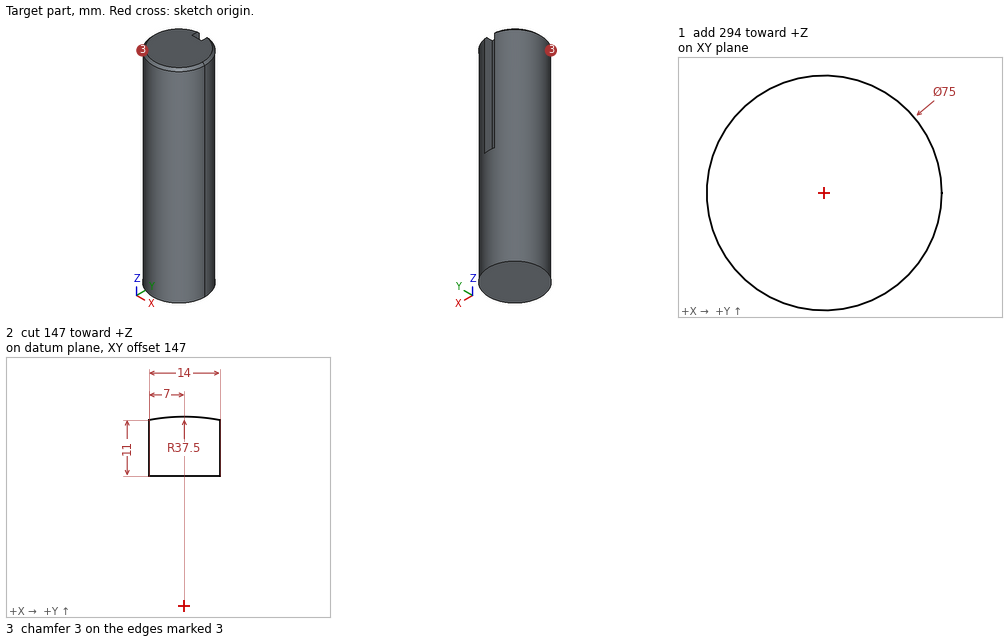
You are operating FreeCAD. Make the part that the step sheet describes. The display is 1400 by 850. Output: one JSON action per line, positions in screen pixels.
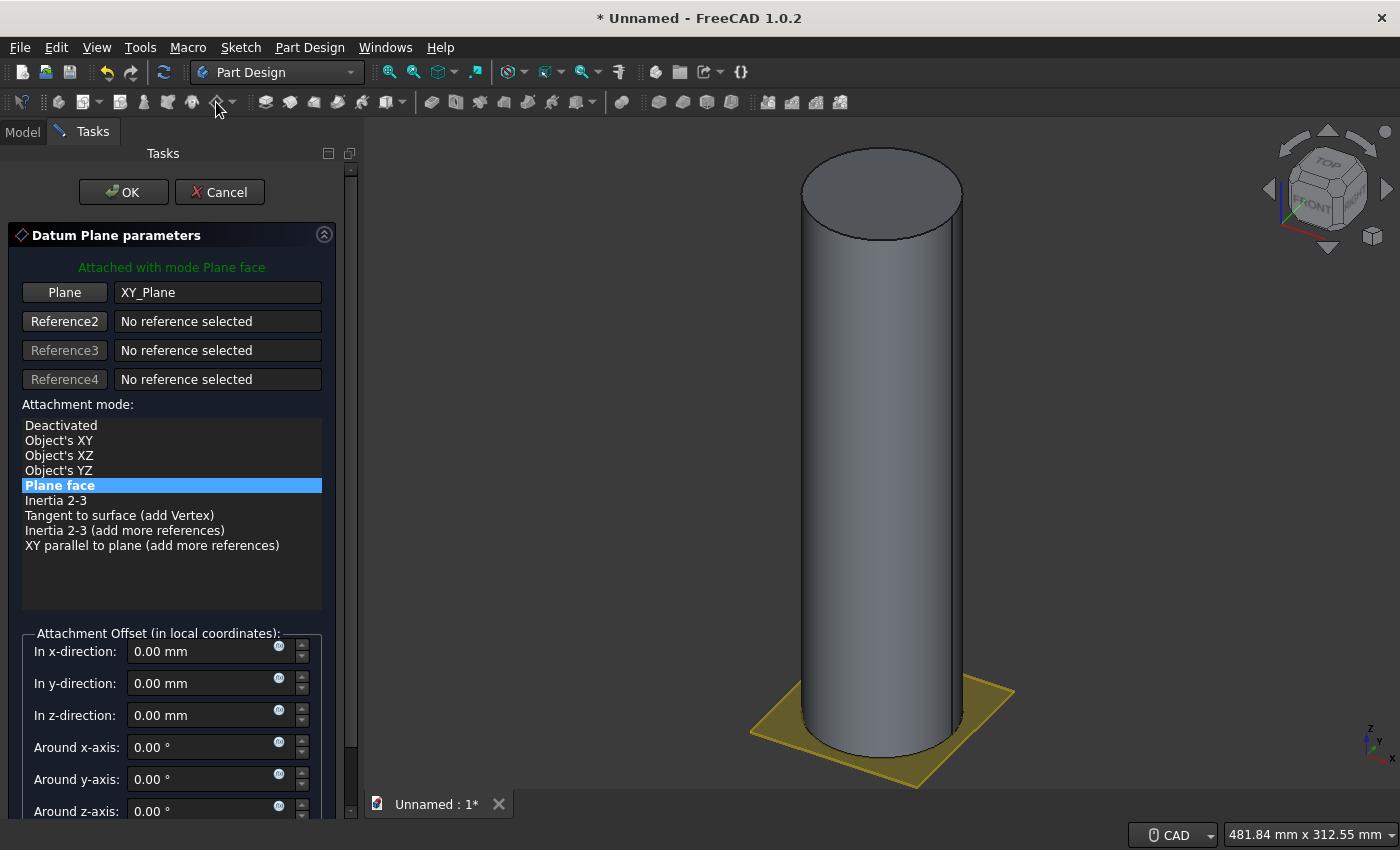
{"action": "triple_click", "coordinate": [210, 715]}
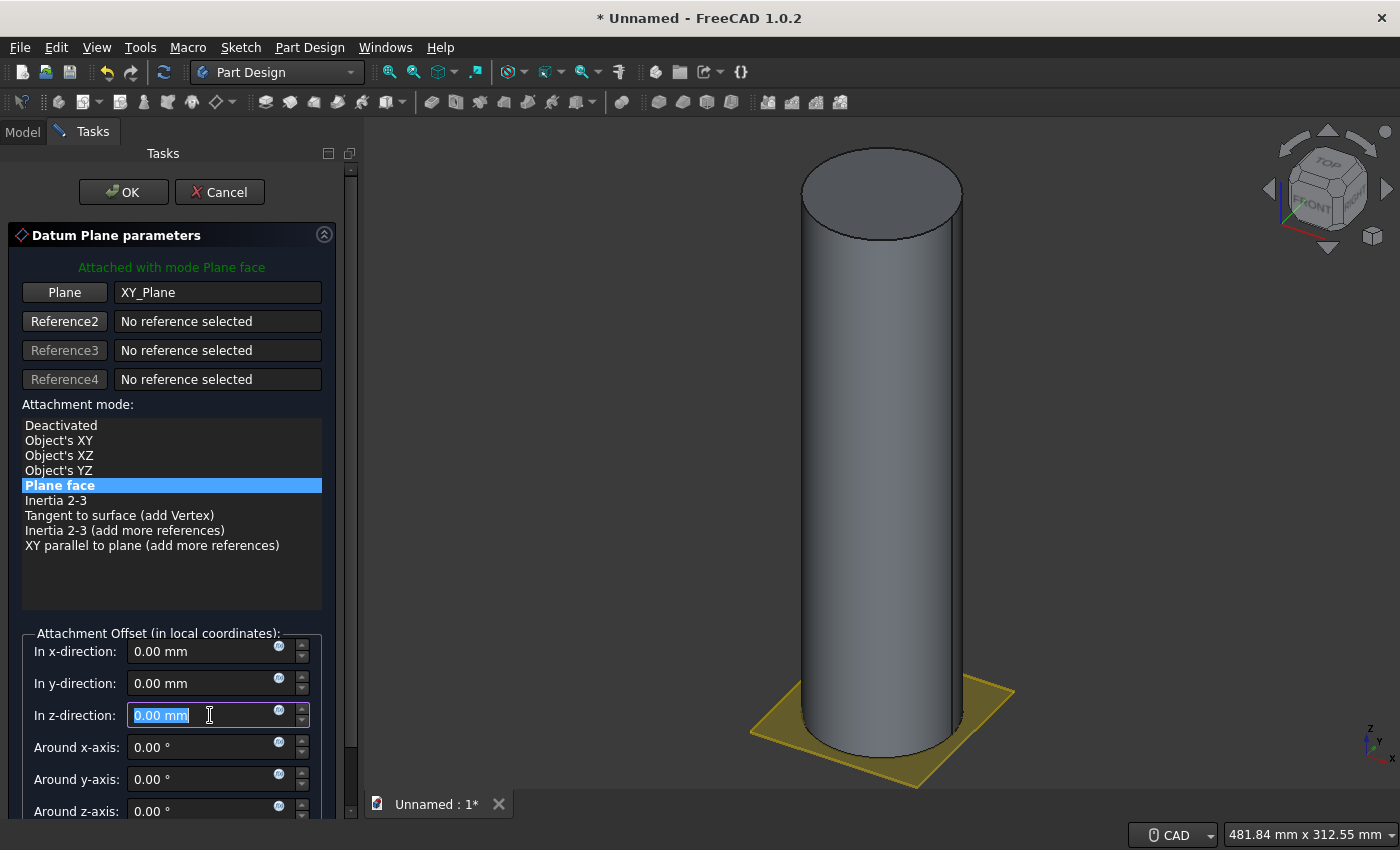
{"action": "type", "text": "147"}
{"action": "key", "text": "Tab"}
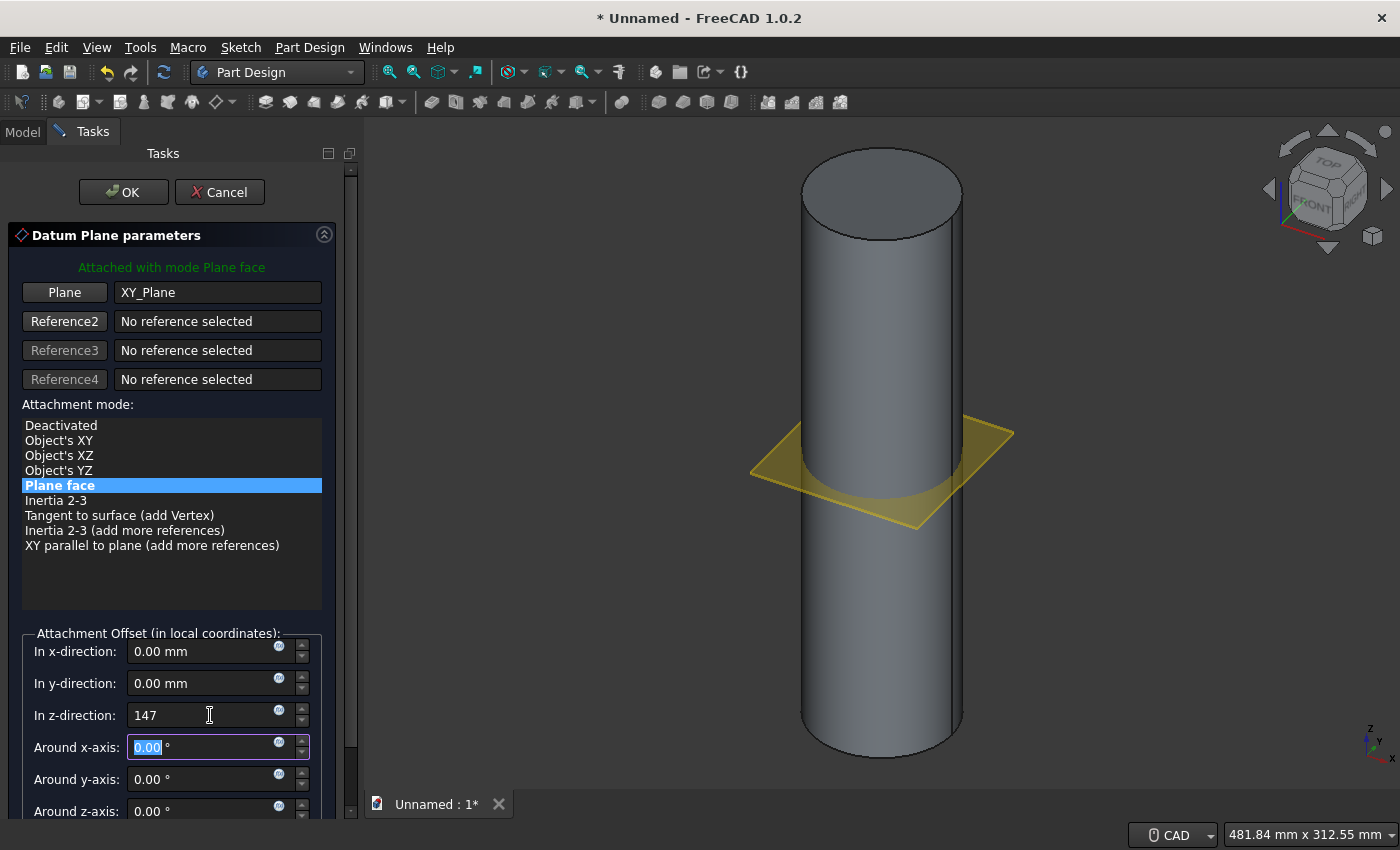
{"action": "left_click", "coordinate": [124, 192]}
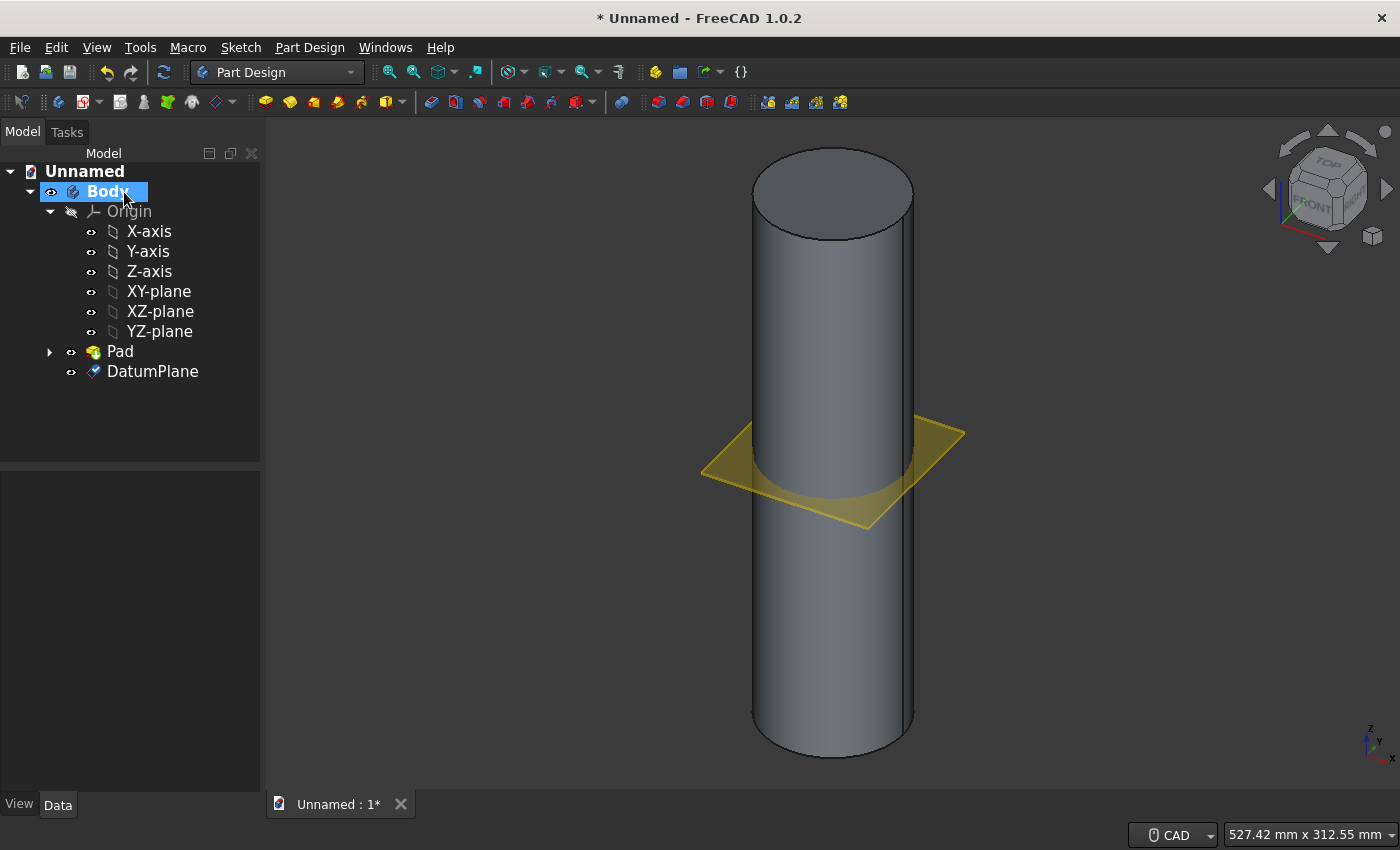
{"action": "left_click", "coordinate": [116, 372]}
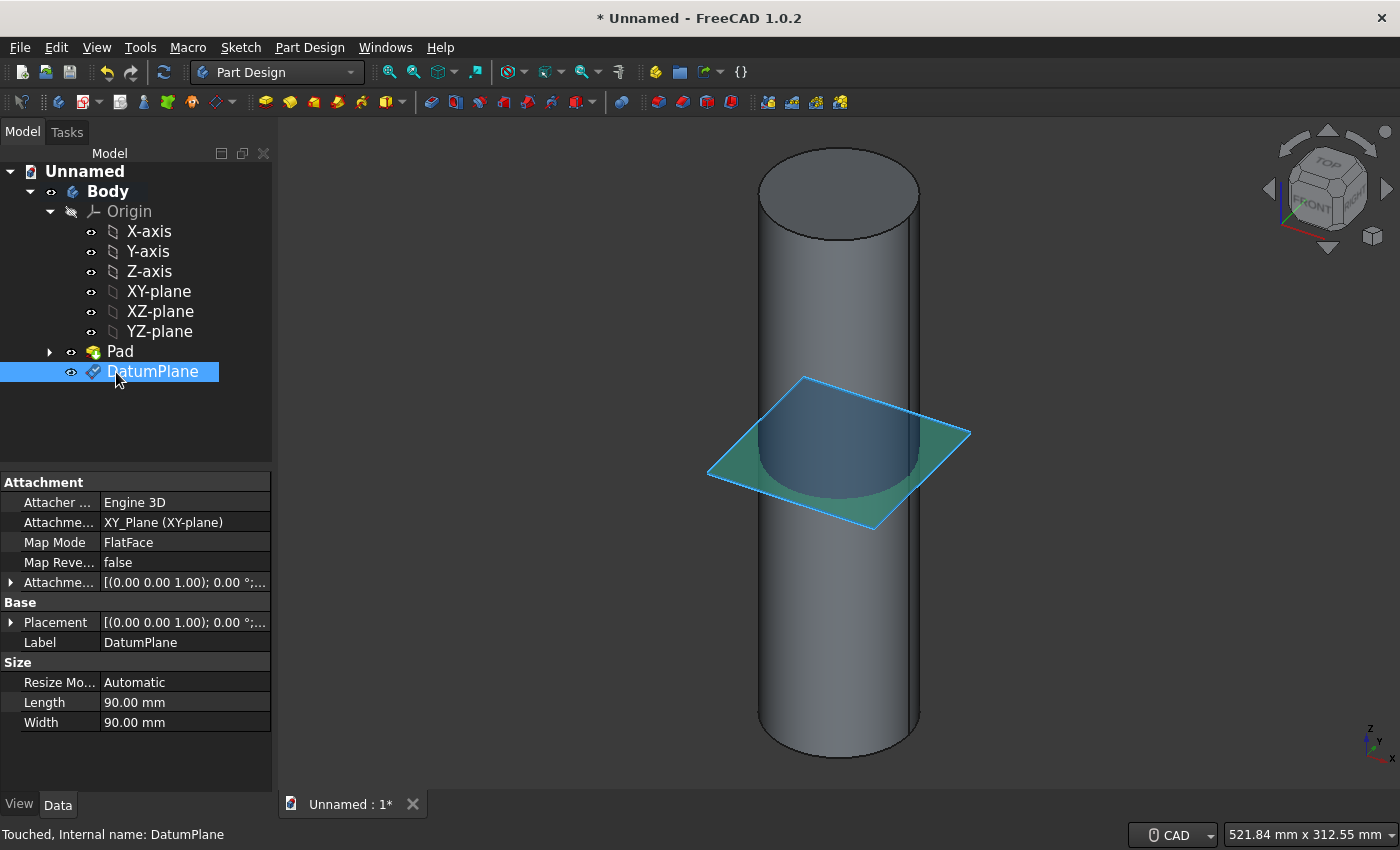
{"action": "left_click", "coordinate": [84, 102]}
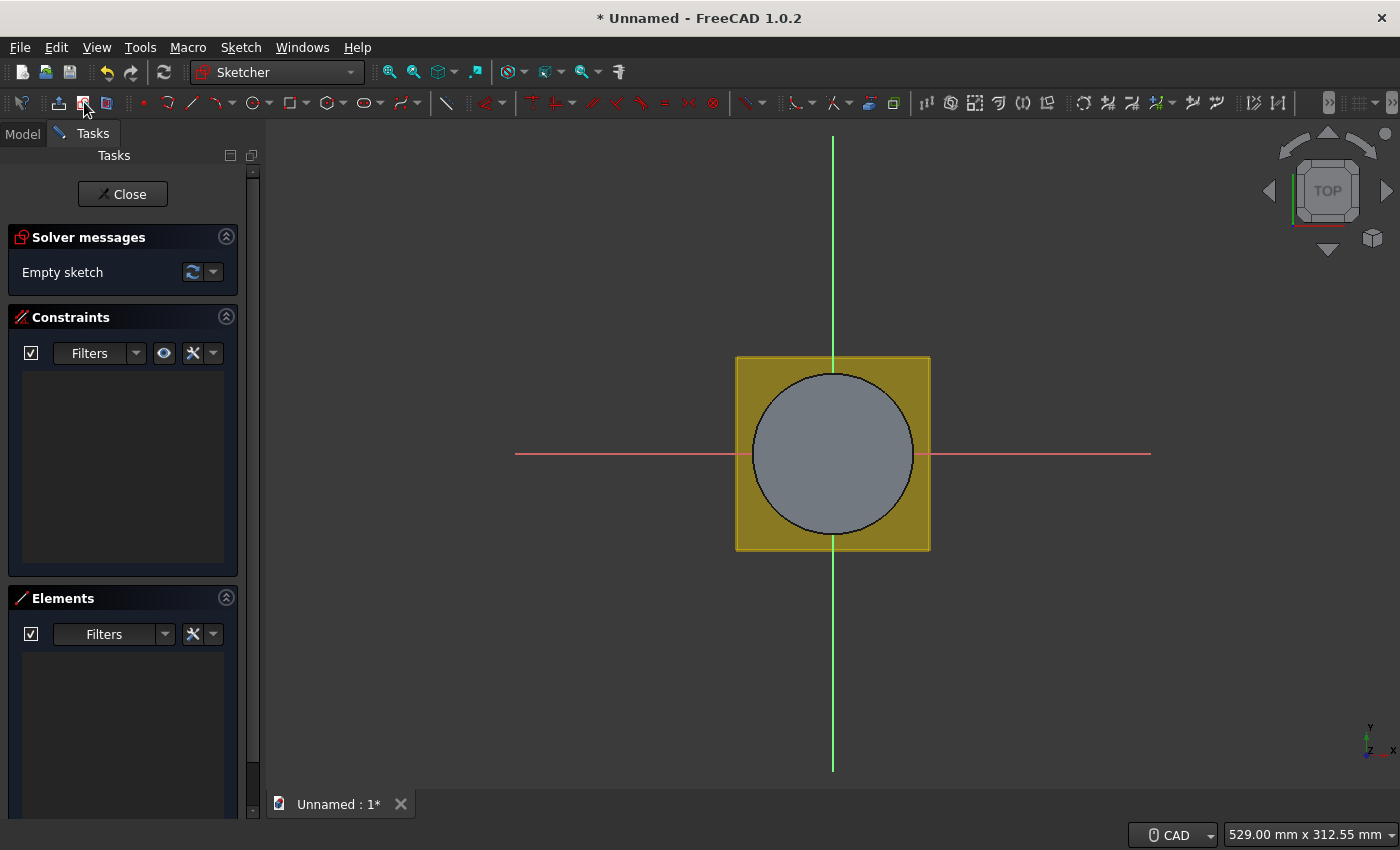
{"action": "key", "text": "q s"}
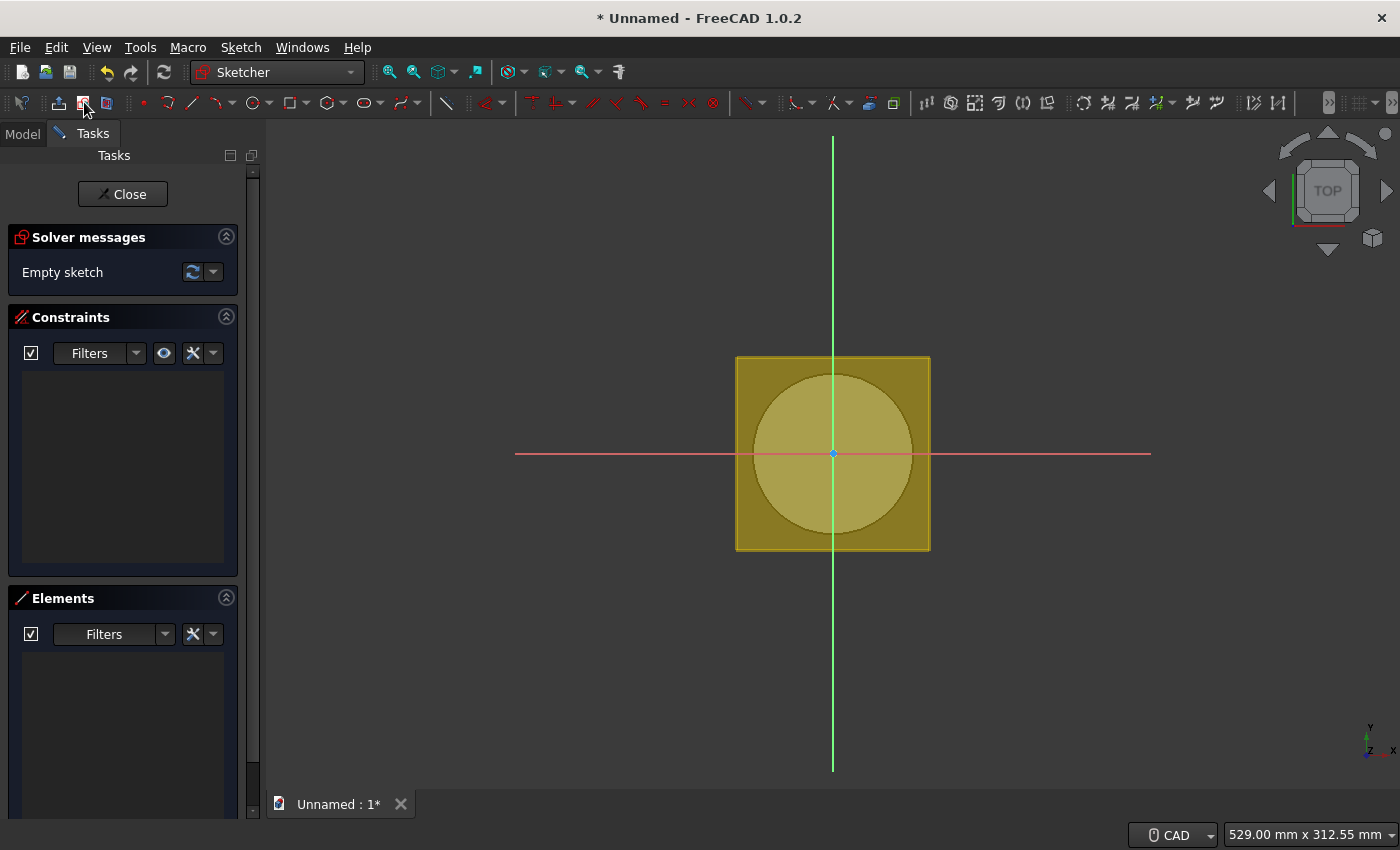
{"action": "scroll", "coordinate": [837, 382], "scroll_direction": "up", "scroll_amount": 14}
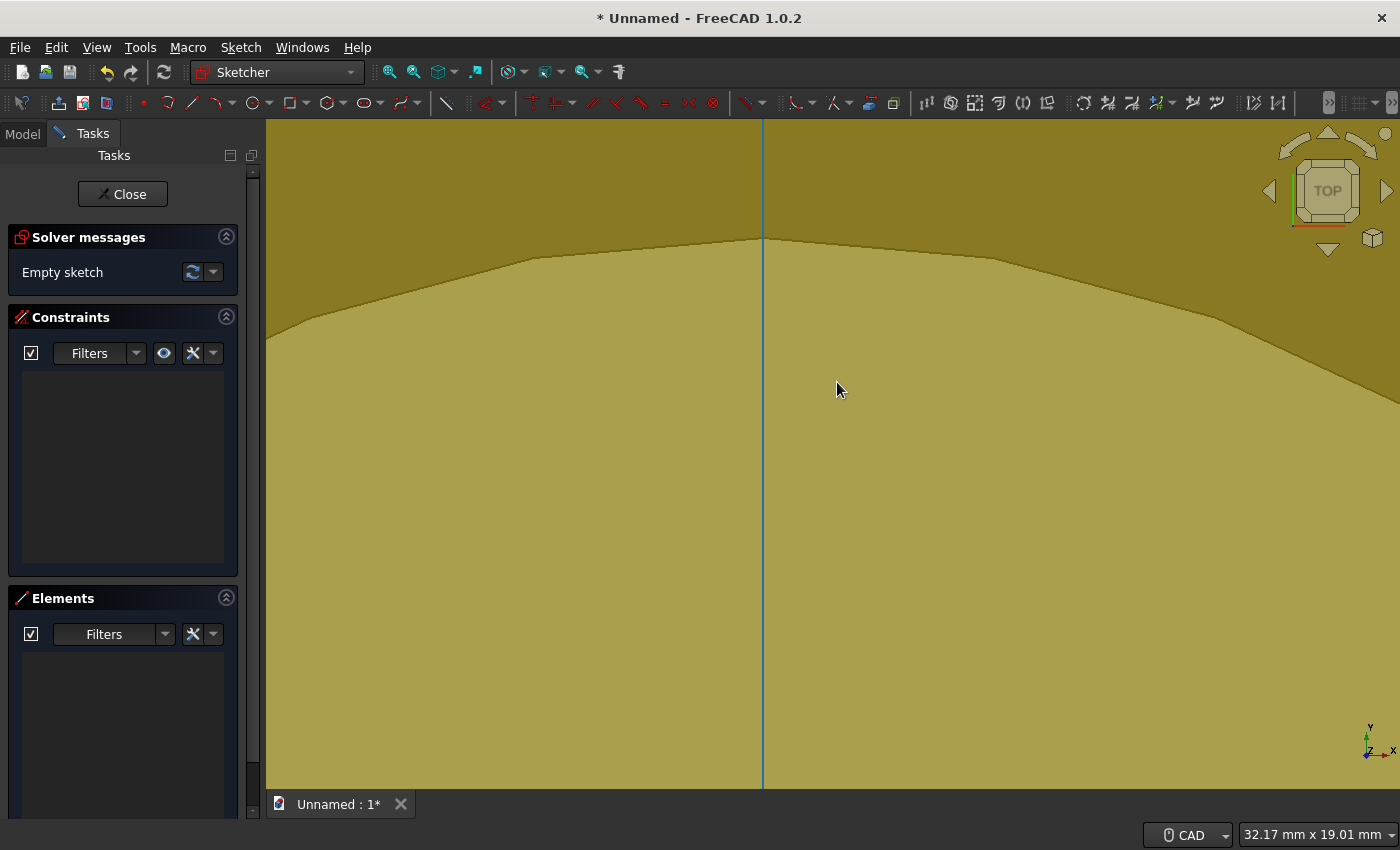
{"action": "left_click", "coordinate": [168, 104]}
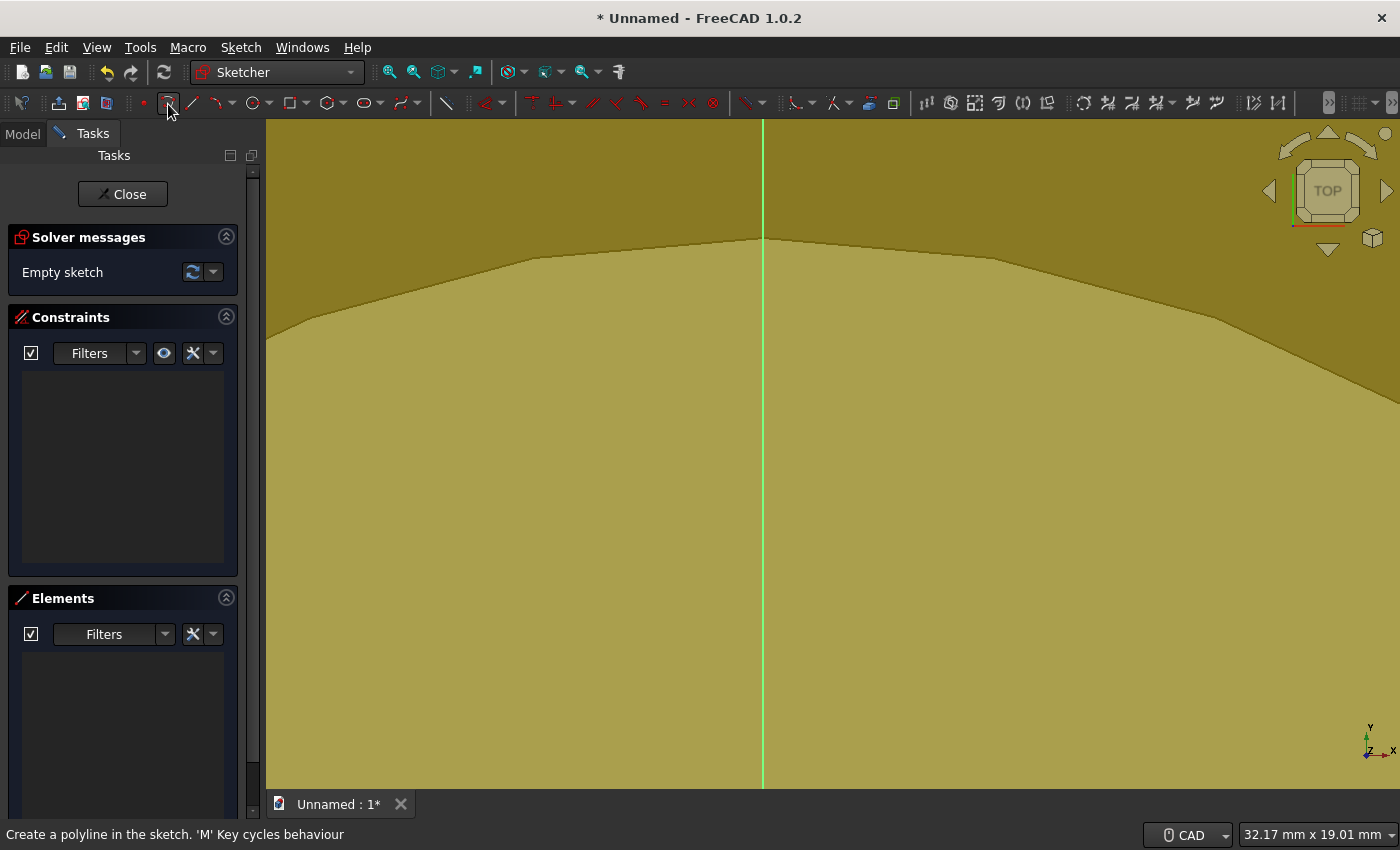
{"action": "left_click", "coordinate": [517, 261]}
{"action": "left_click", "coordinate": [517, 649]}
{"action": "left_click", "coordinate": [1010, 649]}
{"action": "left_click", "coordinate": [1010, 261]}
{"action": "right_click", "coordinate": [1010, 261]}